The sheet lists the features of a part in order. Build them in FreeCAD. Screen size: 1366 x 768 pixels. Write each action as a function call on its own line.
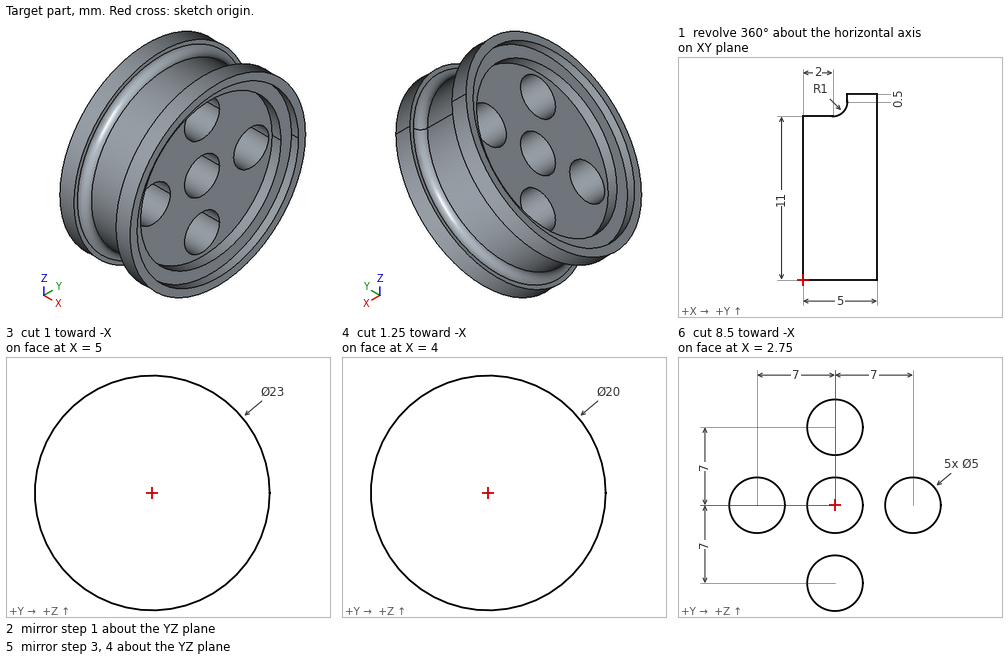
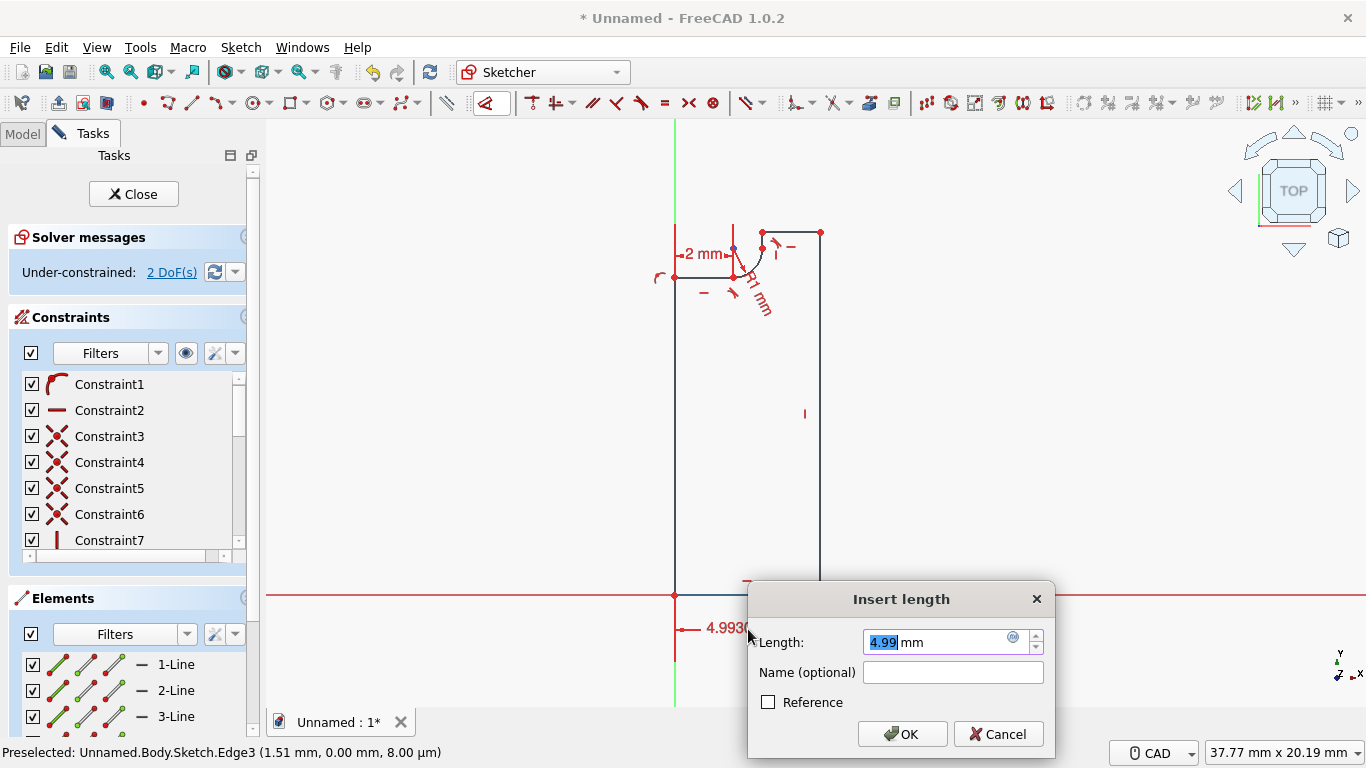
text(5)
key(Return)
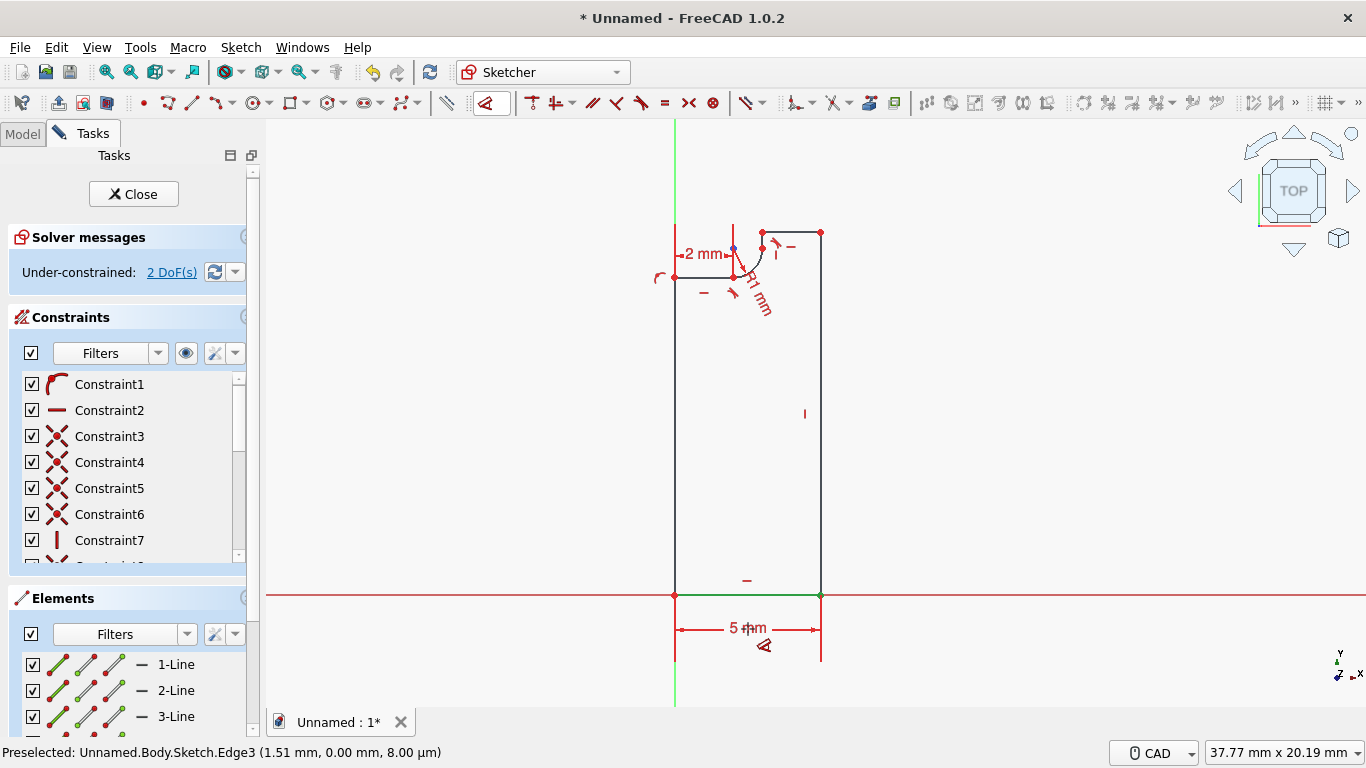
click(675, 373)
click(641, 436)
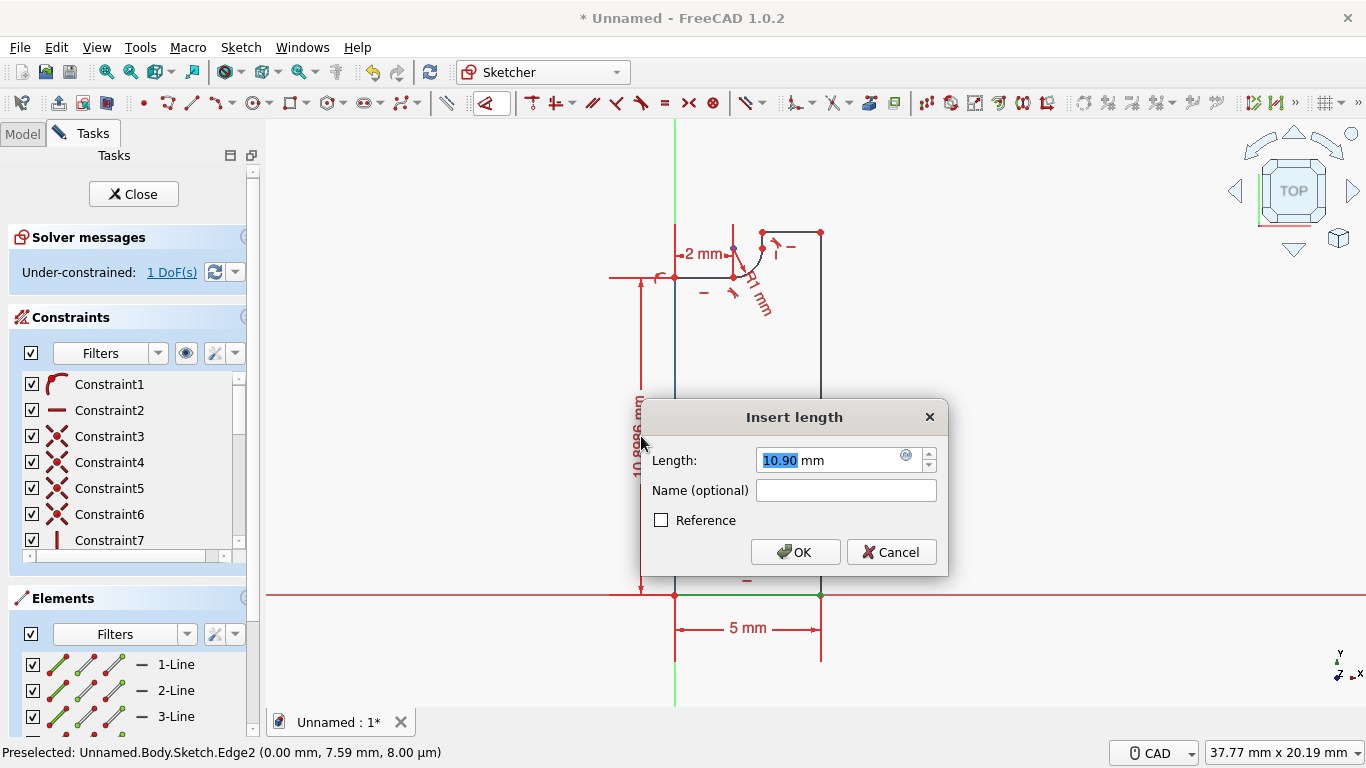
text(11)
key(Return)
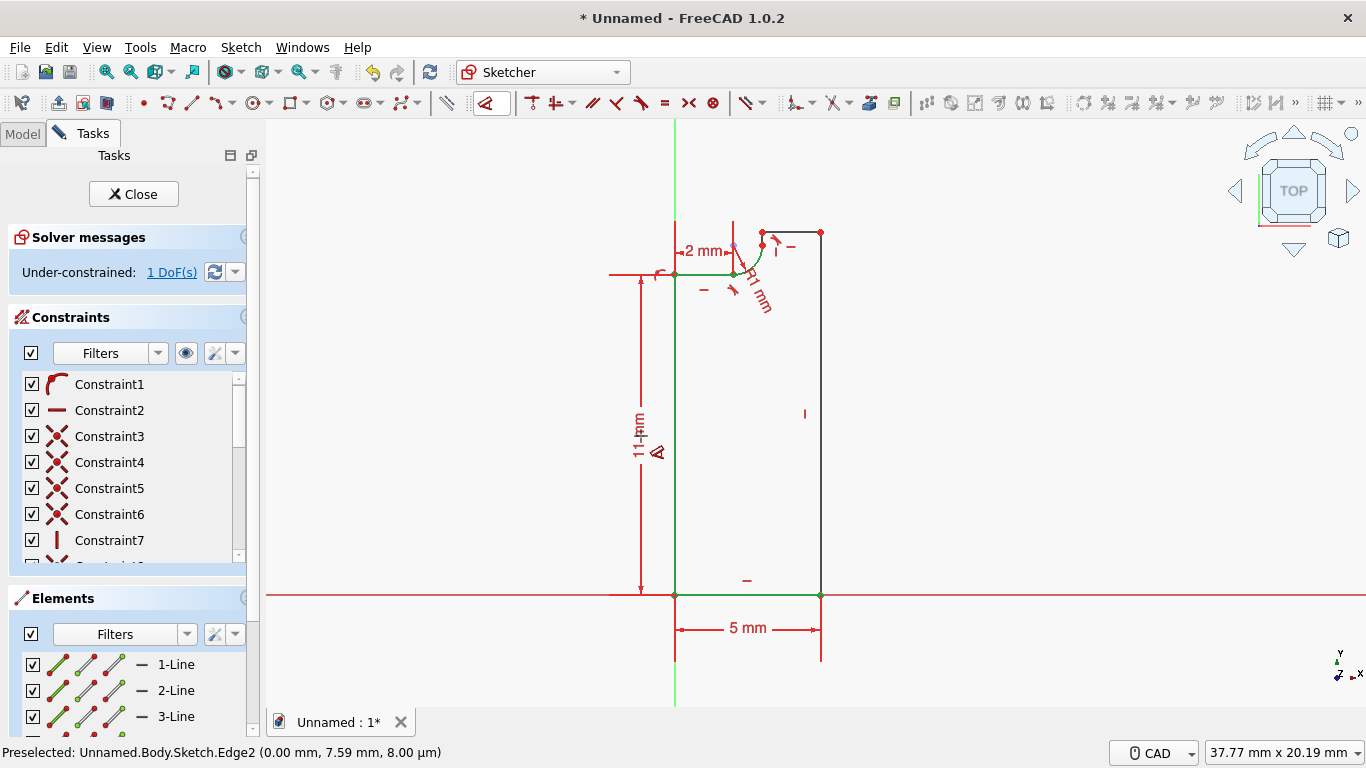
scroll(762, 239, up, 6)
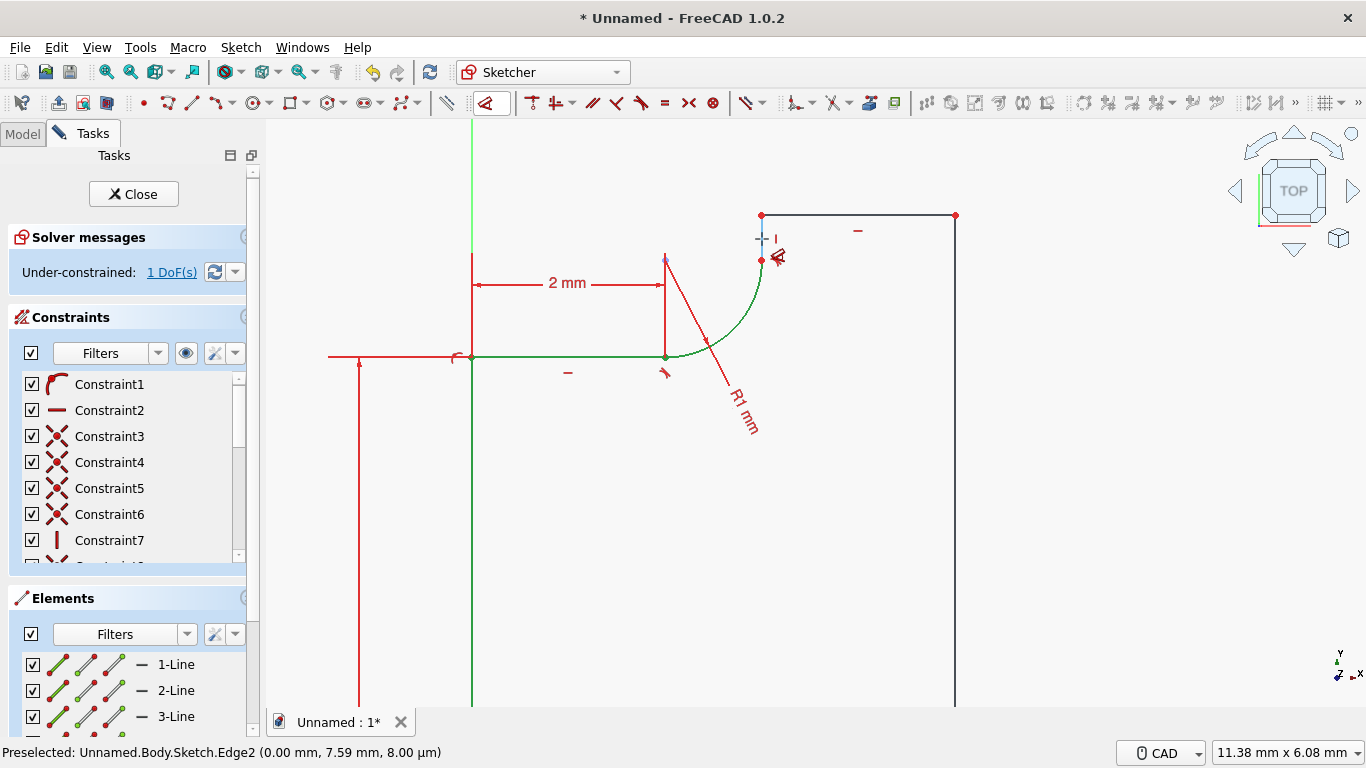
click(762, 238)
click(796, 238)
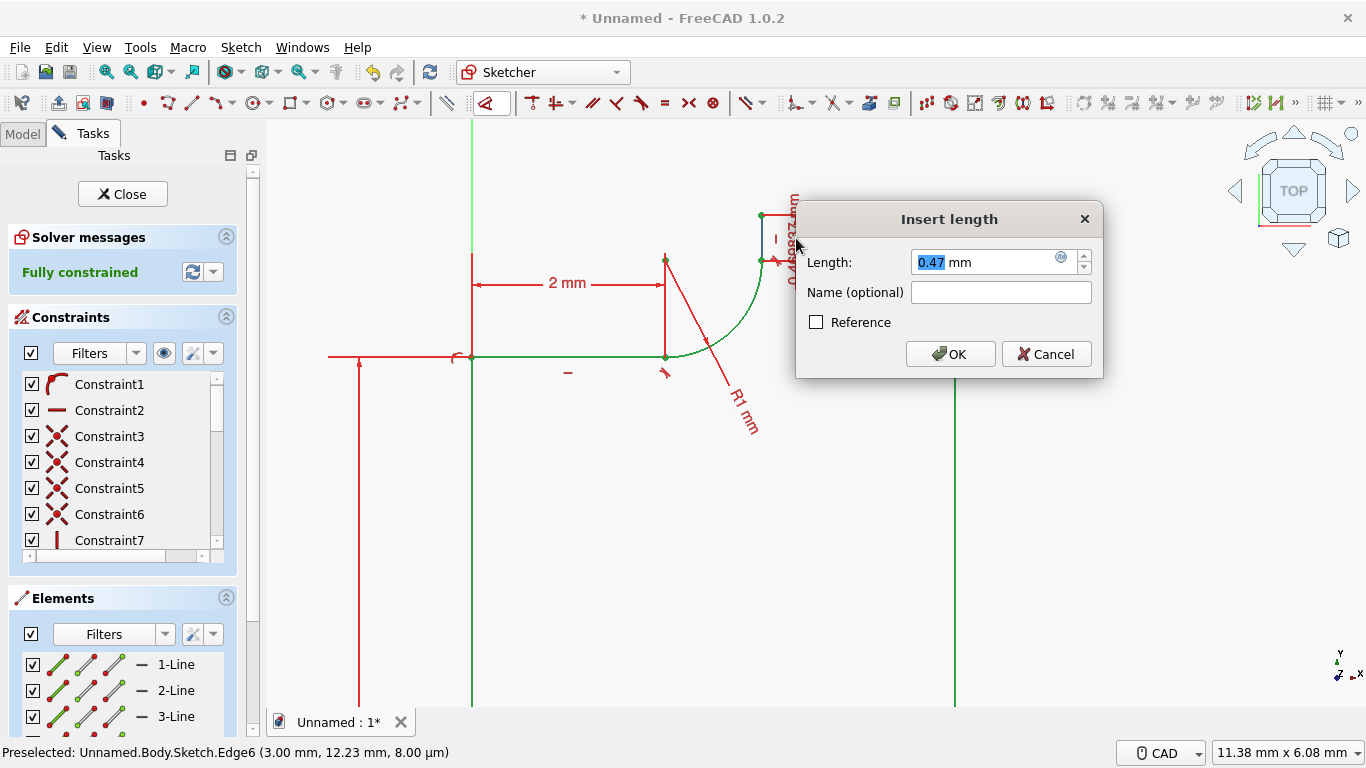
text(0.5)
key(Return)
key(Escape)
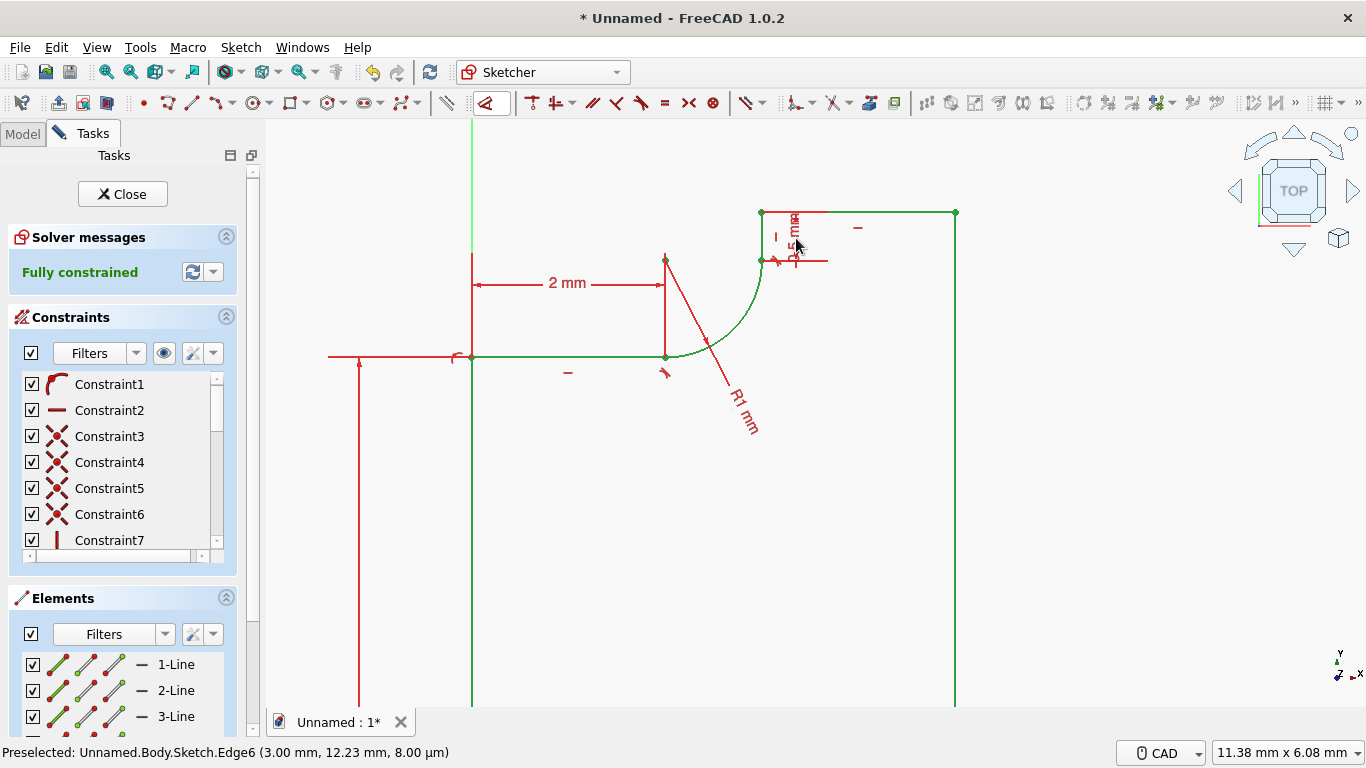
click(123, 194)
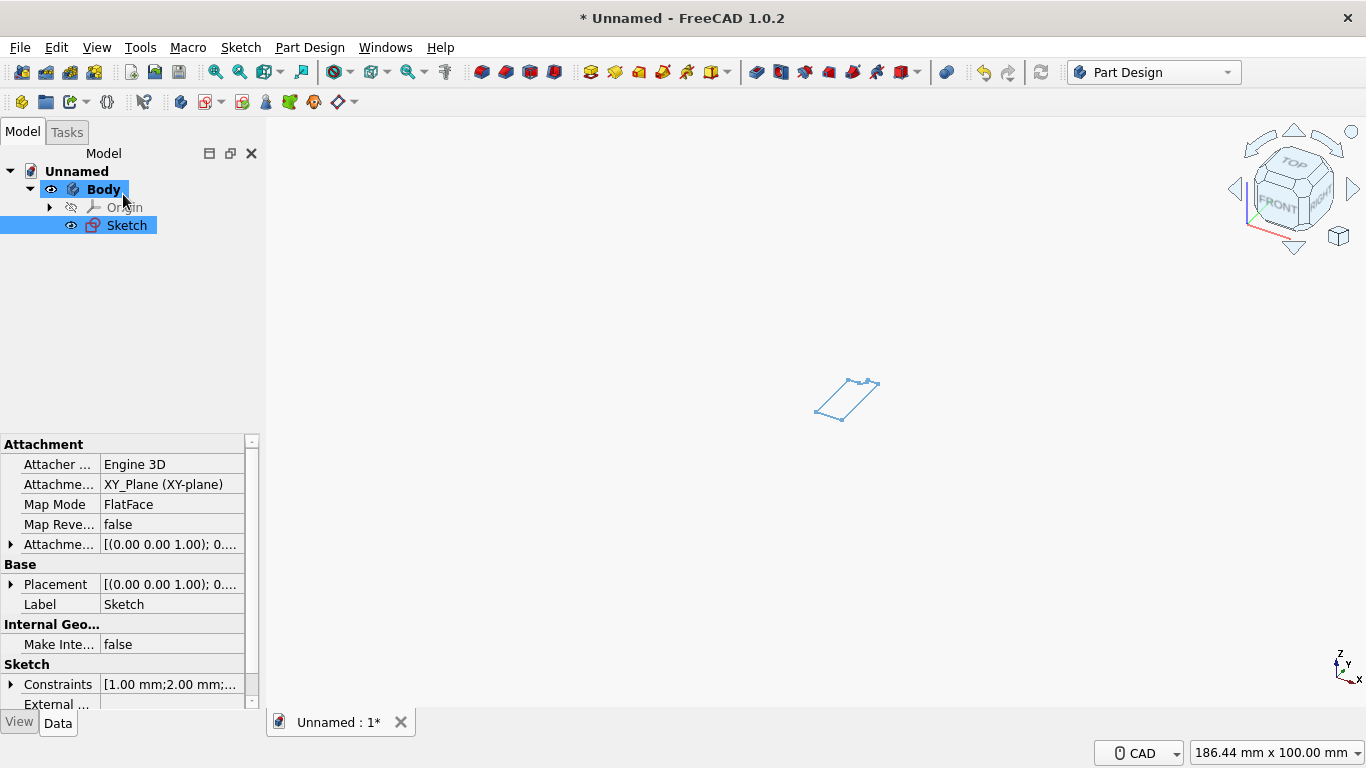
click(616, 72)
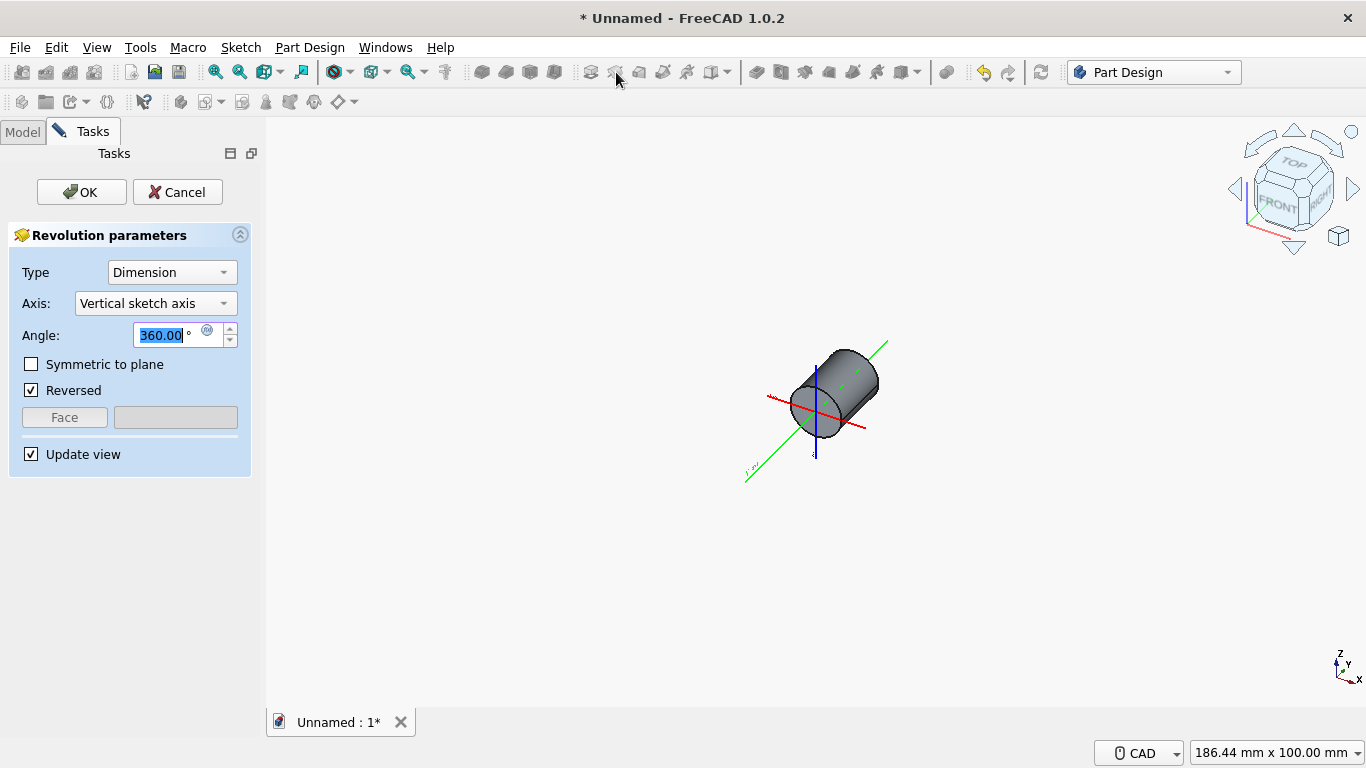
click(156, 304)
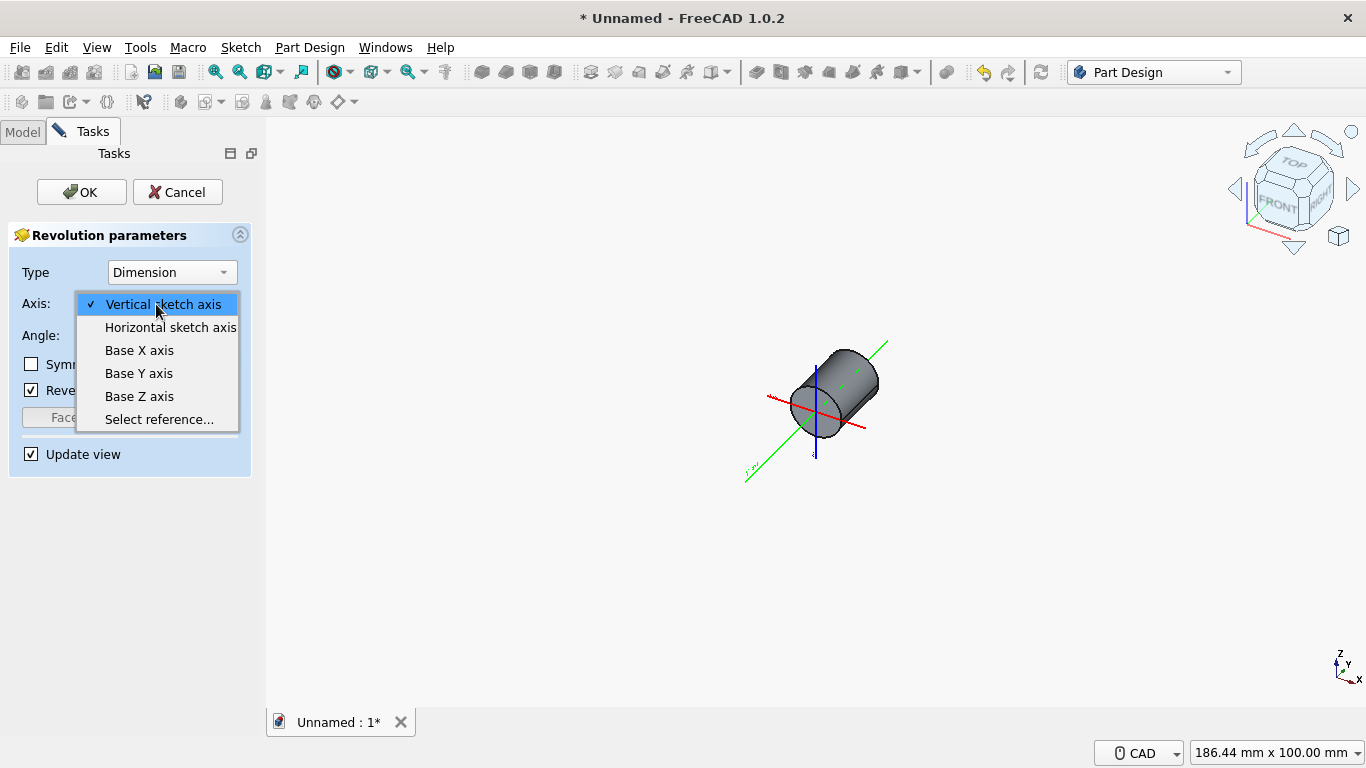
click(156, 328)